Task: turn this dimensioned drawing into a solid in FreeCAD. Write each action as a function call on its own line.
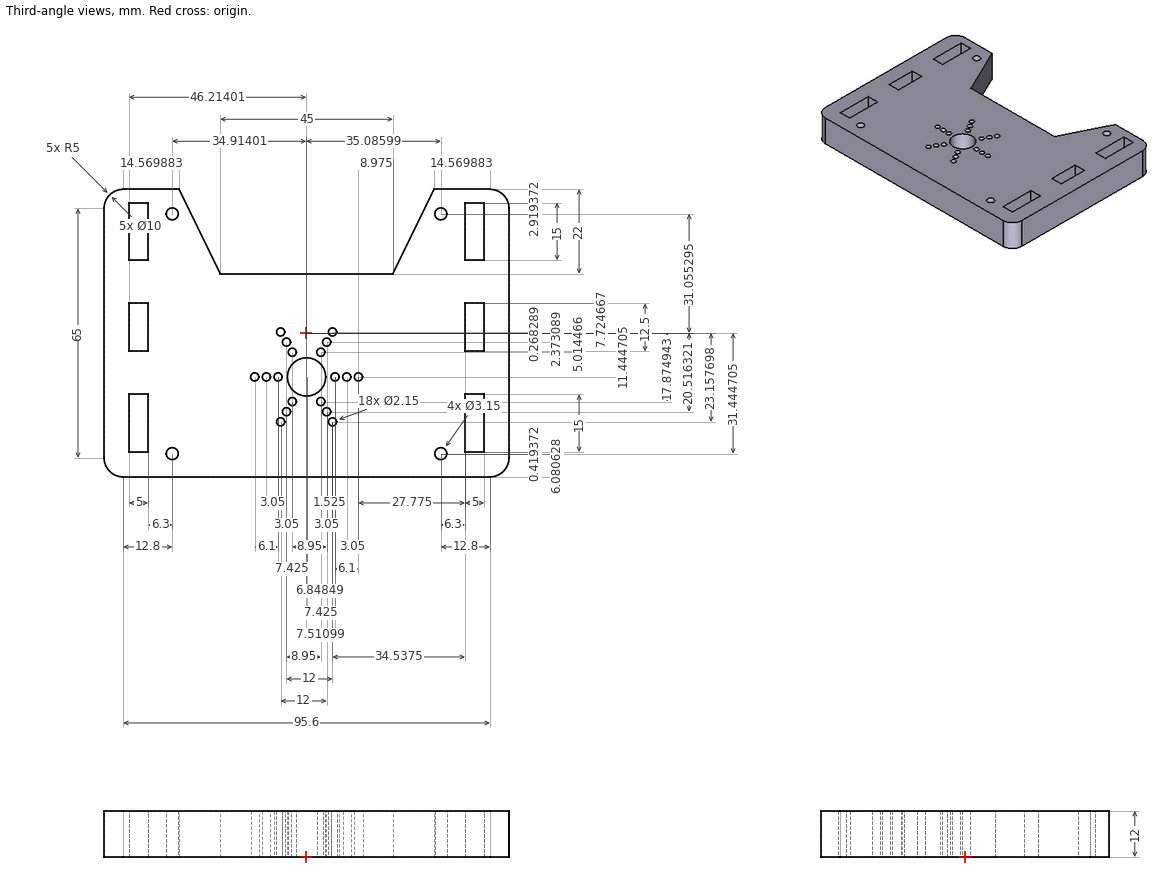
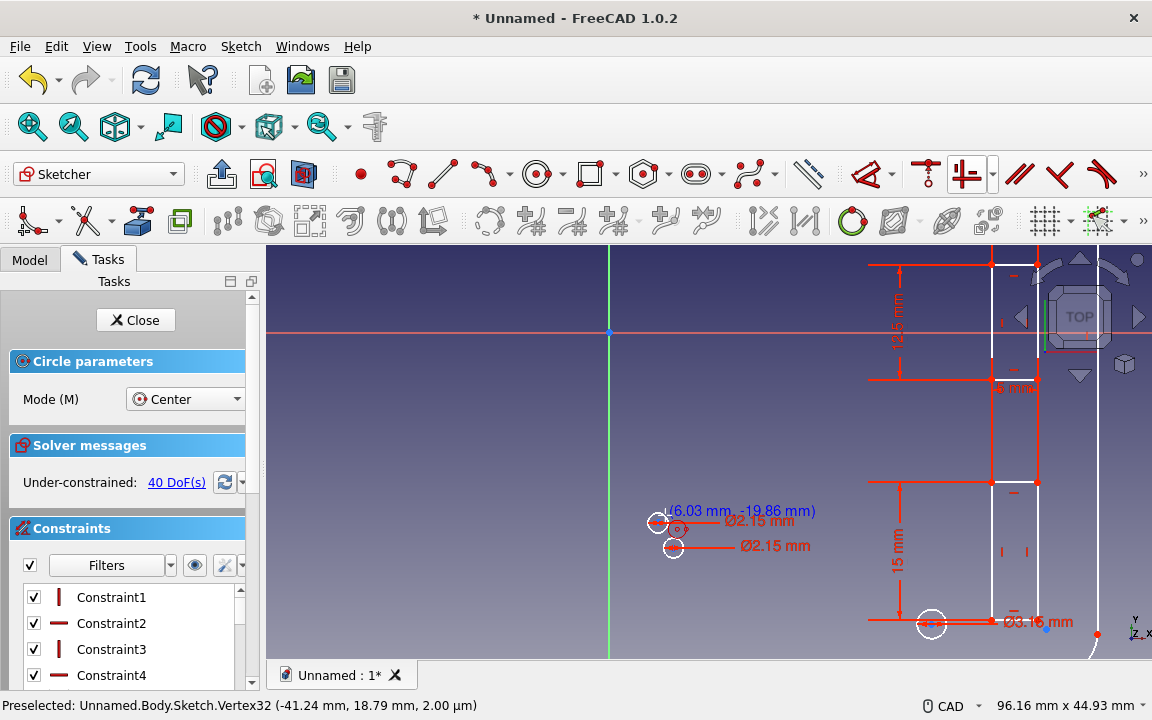
scroll(644, 498, up, 5)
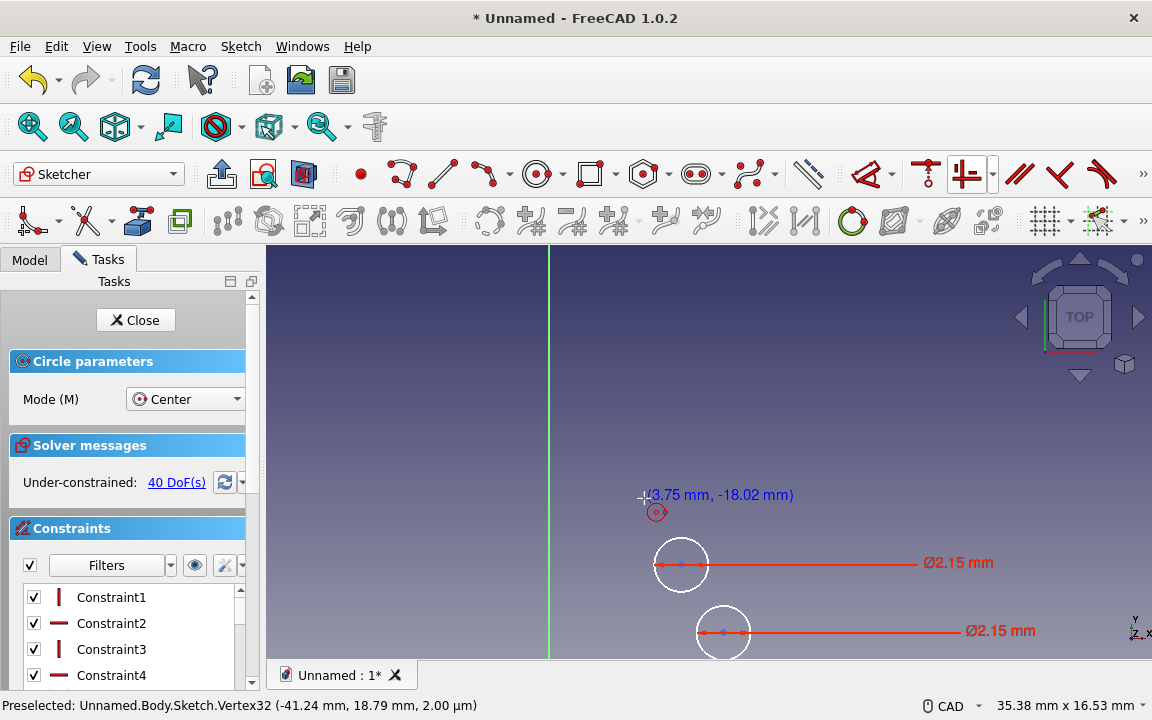
scroll(654, 515, down, 10)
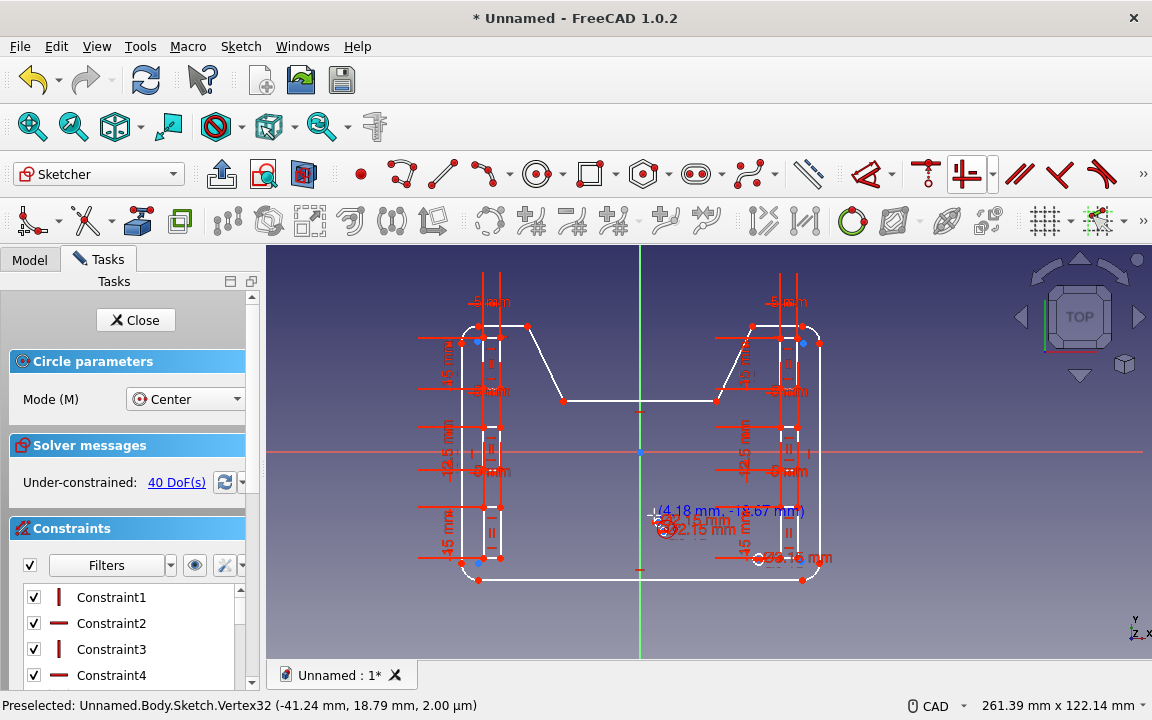
scroll(653, 513, up, 5)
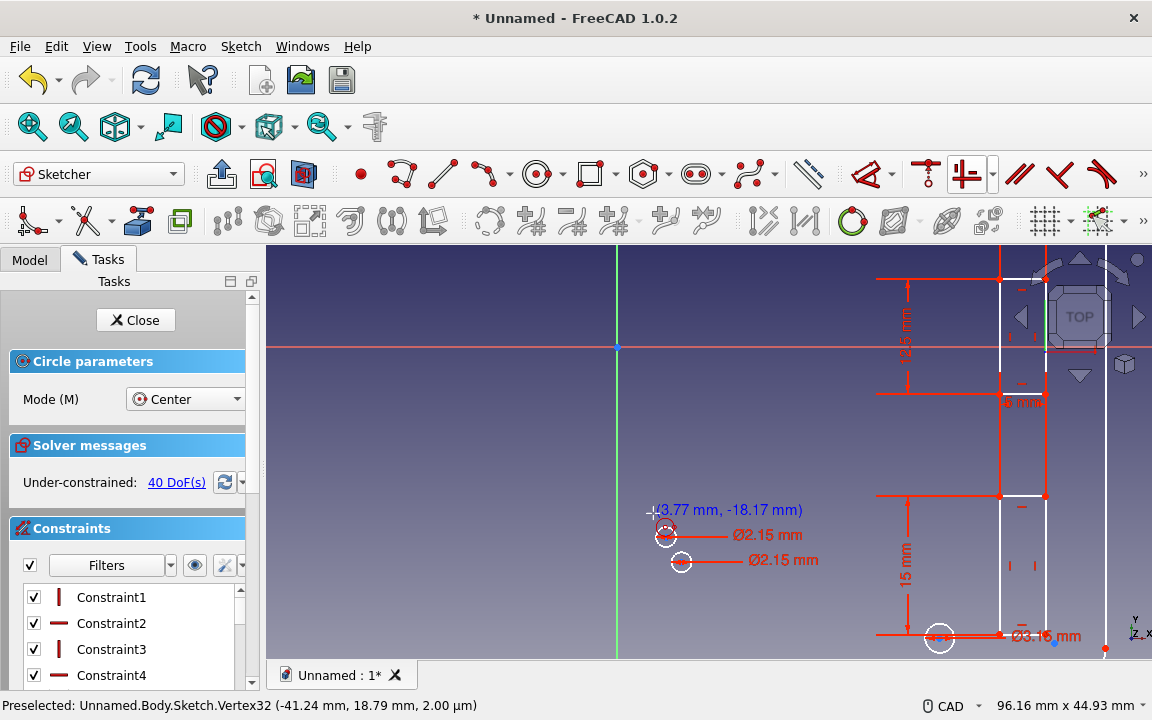
click(652, 512)
move(659, 505)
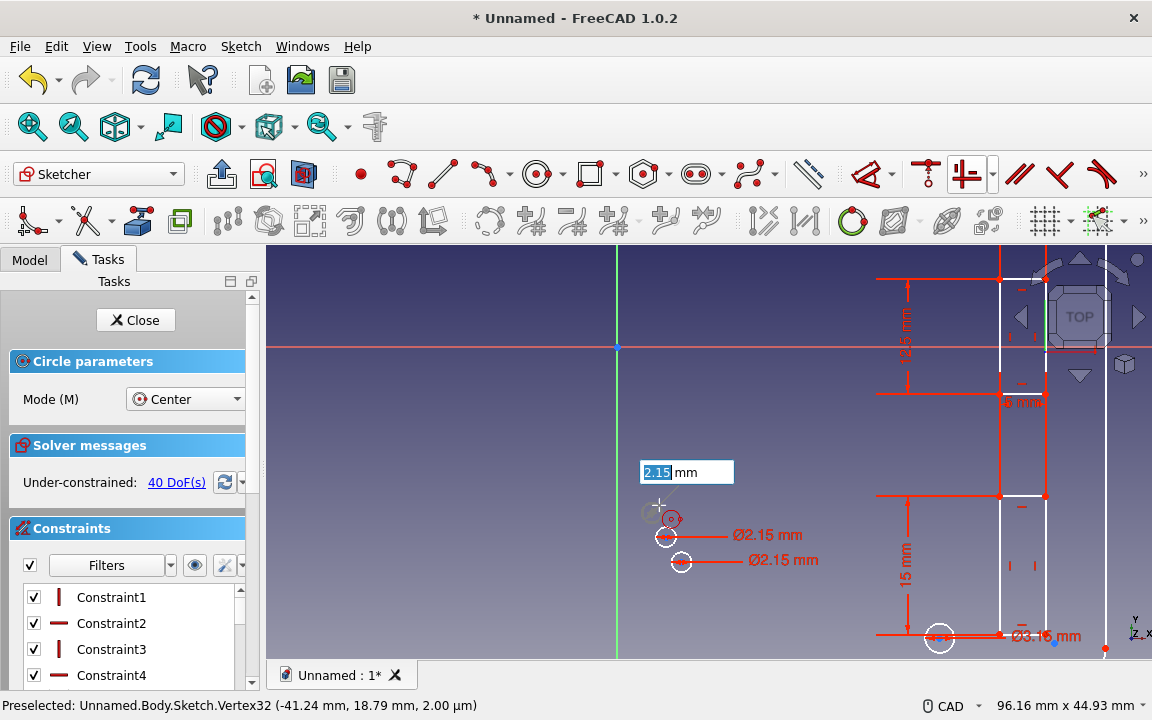
text(2.15)
key(Return)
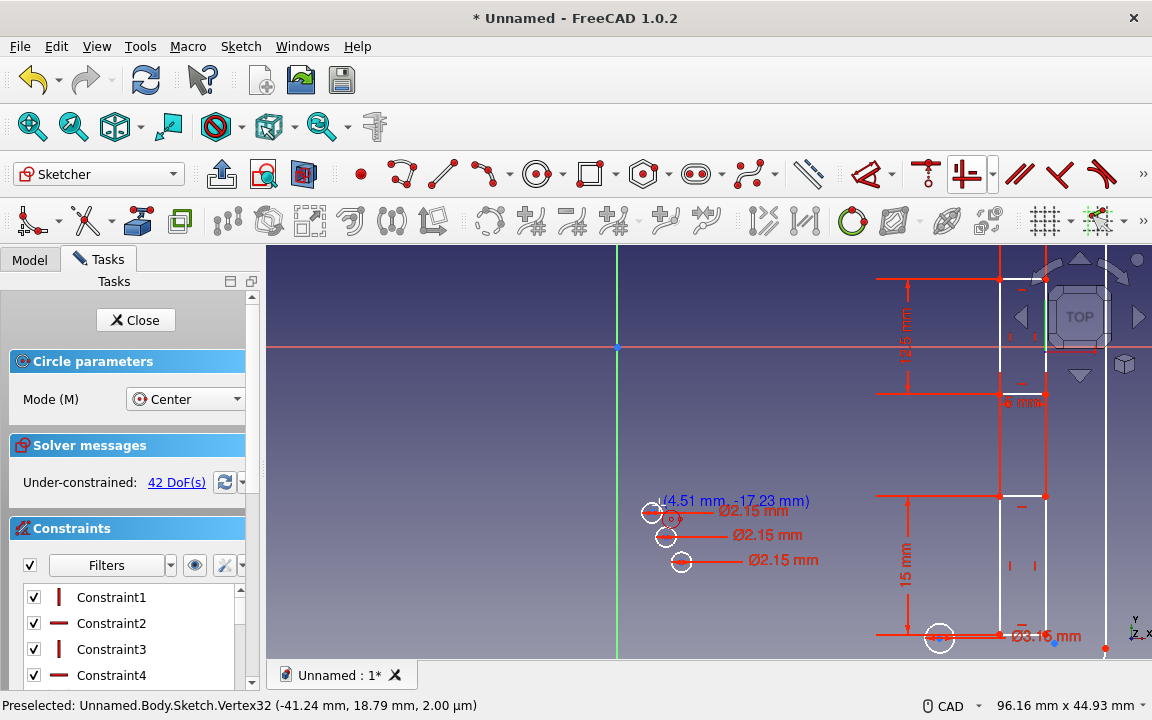
scroll(743, 453, up, 5)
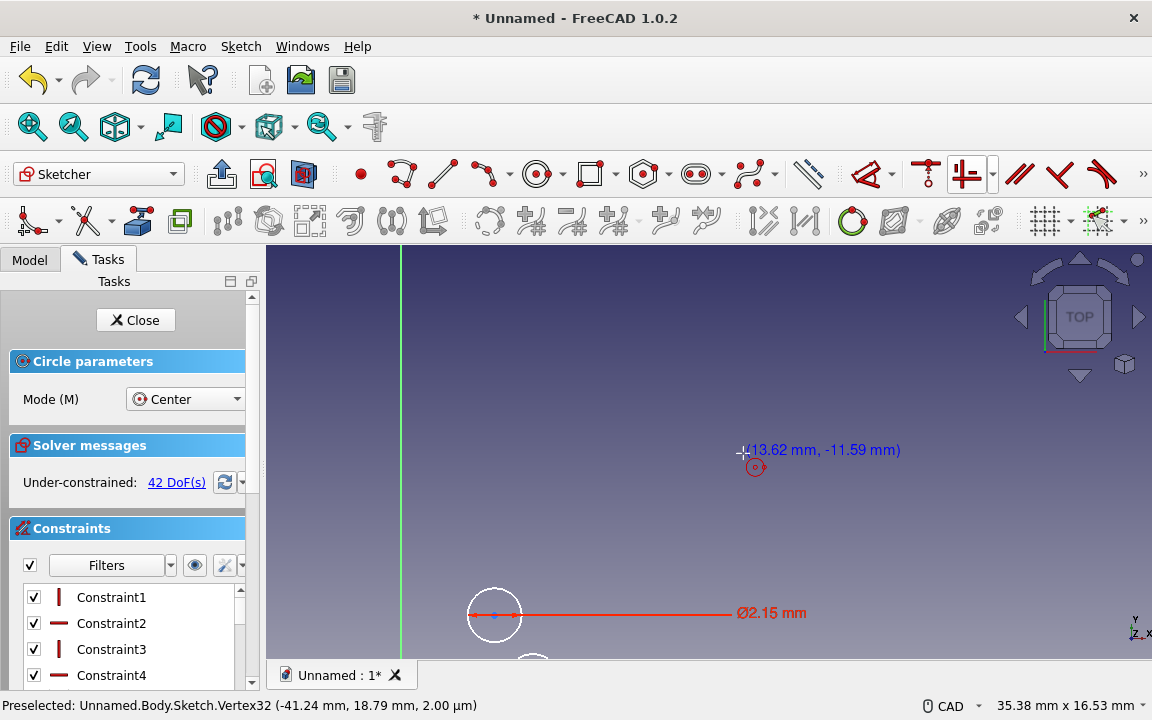
scroll(678, 497, down, 10)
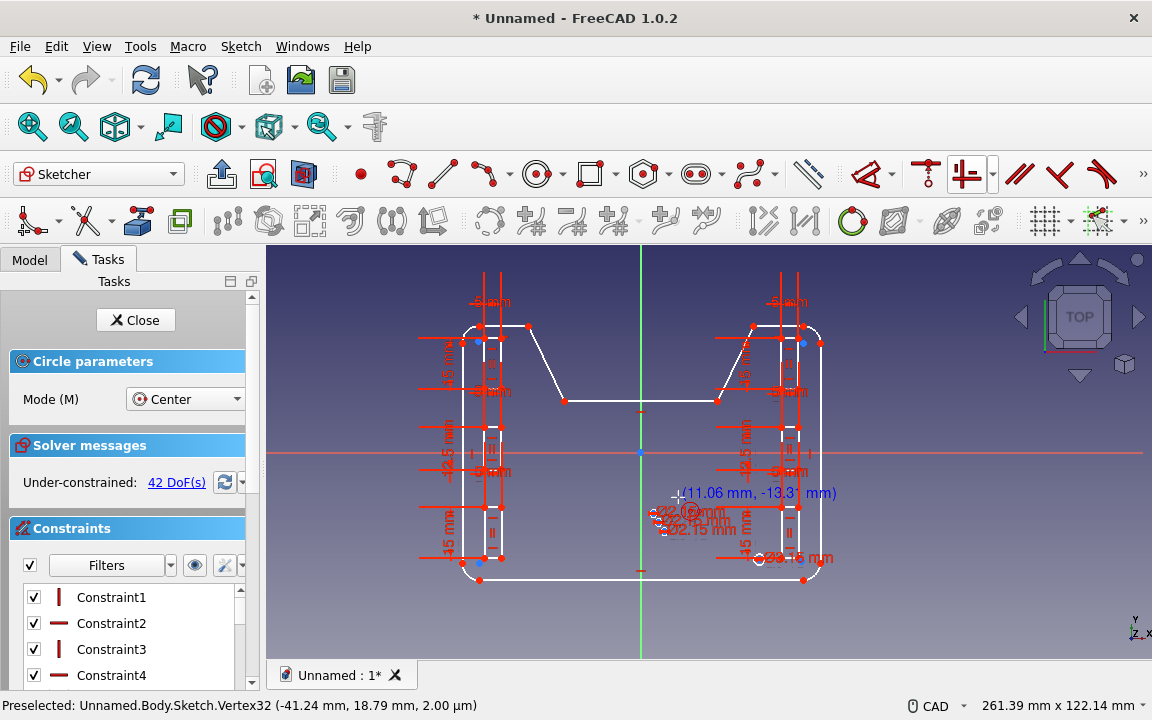
click(687, 491)
move(690, 489)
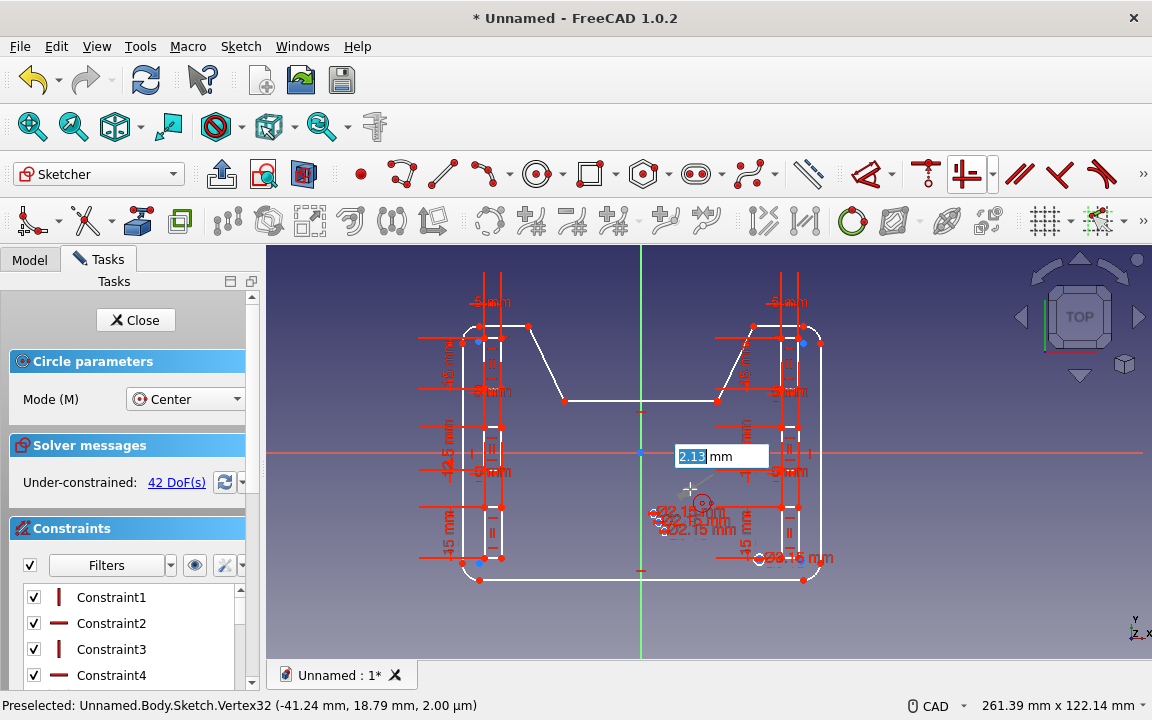
text(2.15)
key(Return)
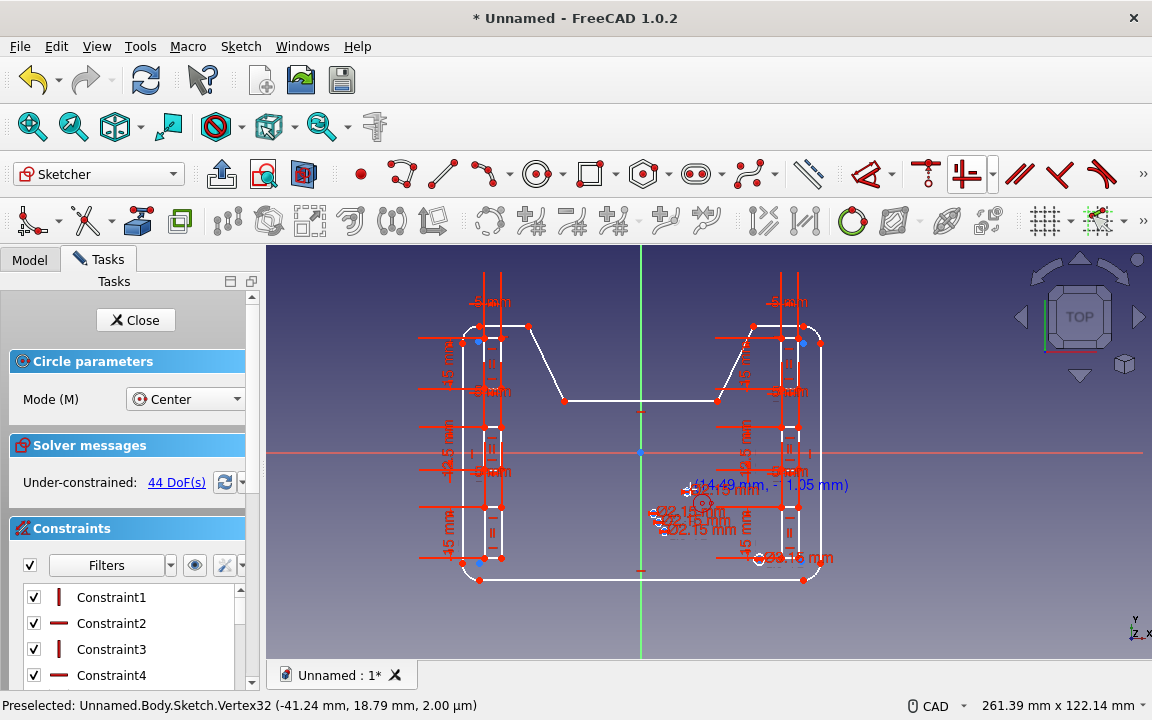
scroll(677, 491, up, 10)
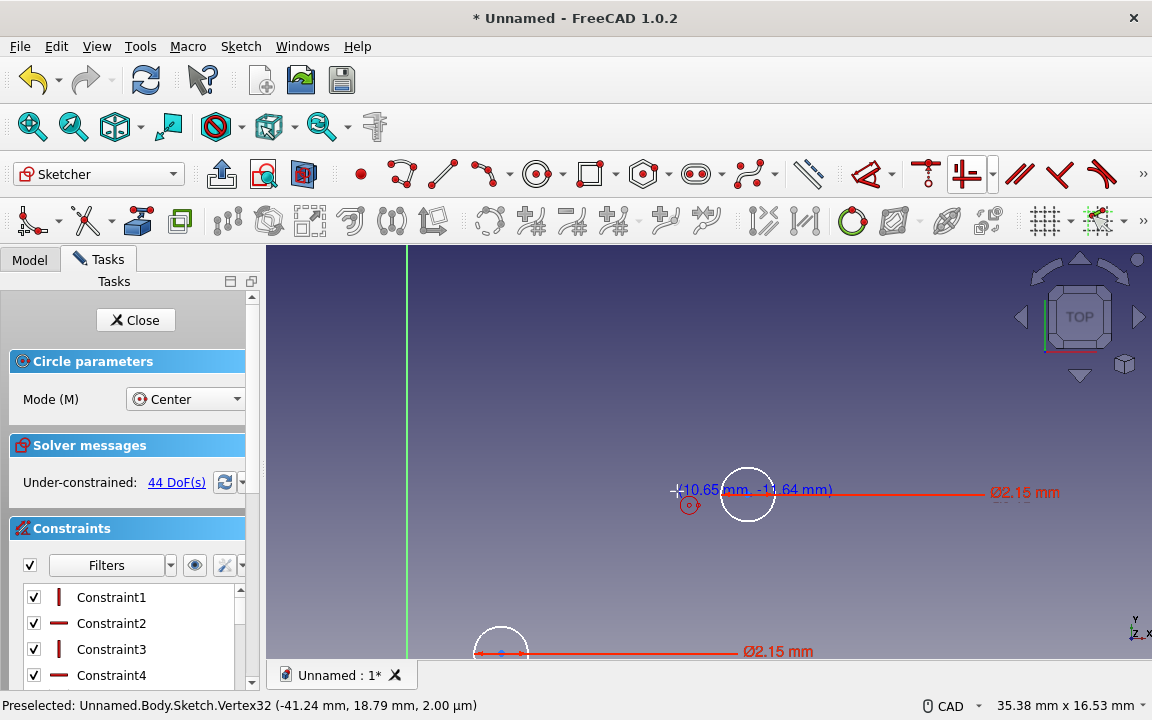
scroll(677, 491, down, 10)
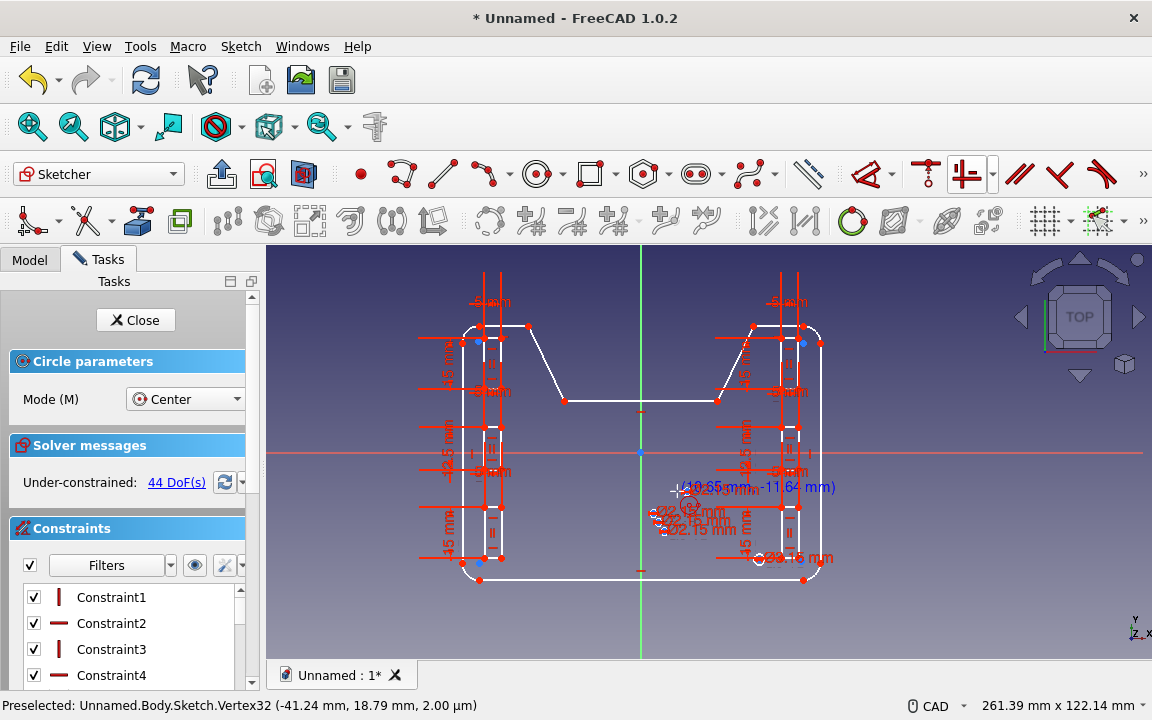
scroll(677, 491, up, 5)